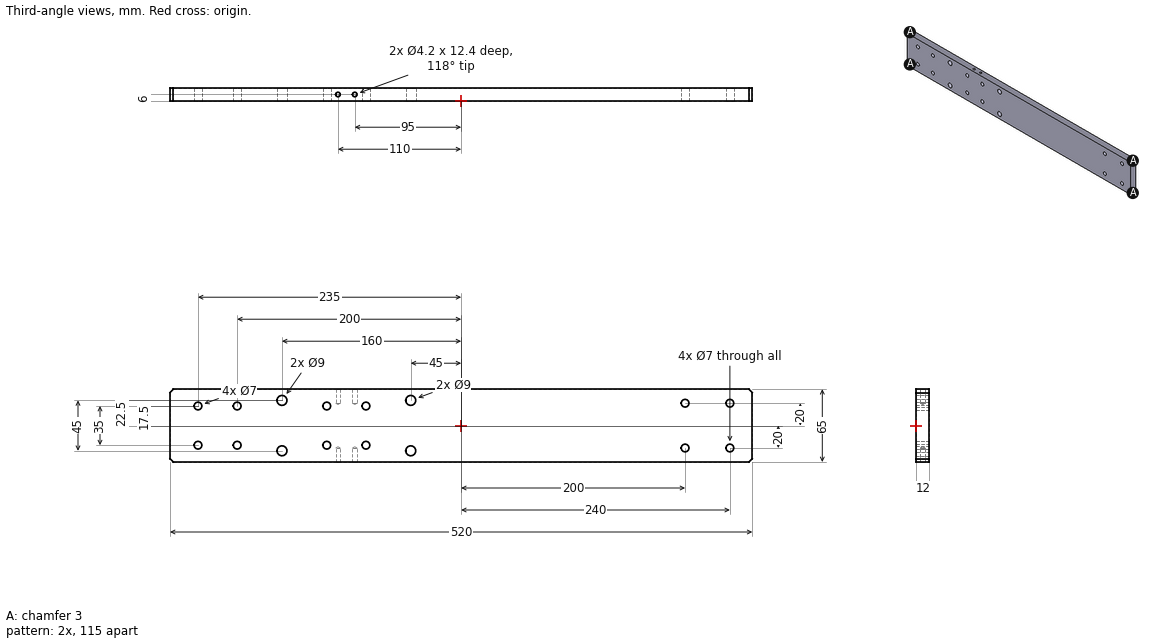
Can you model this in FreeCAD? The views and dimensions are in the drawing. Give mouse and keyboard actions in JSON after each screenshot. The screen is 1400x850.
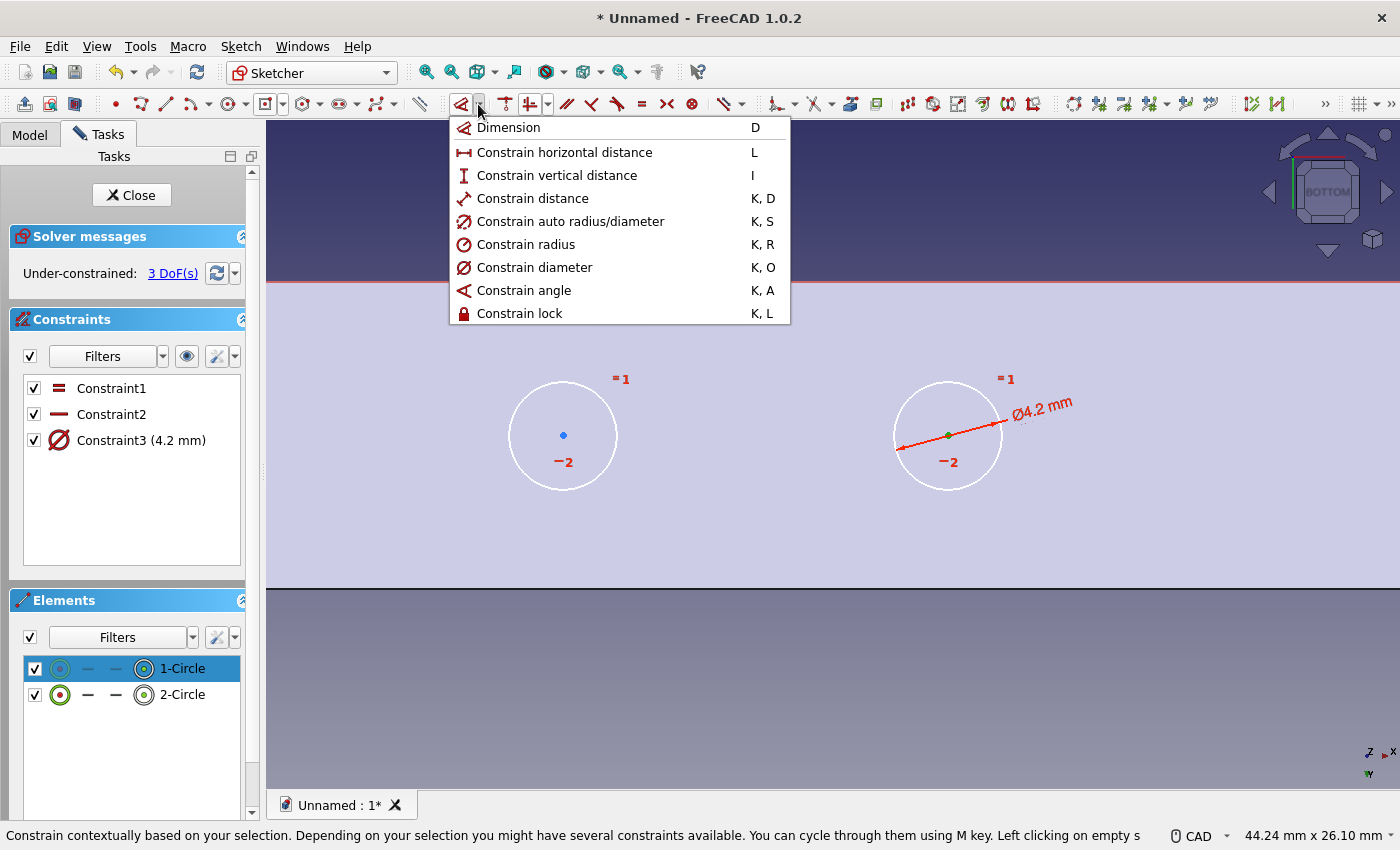
{"action": "left_click", "coordinate": [620, 176]}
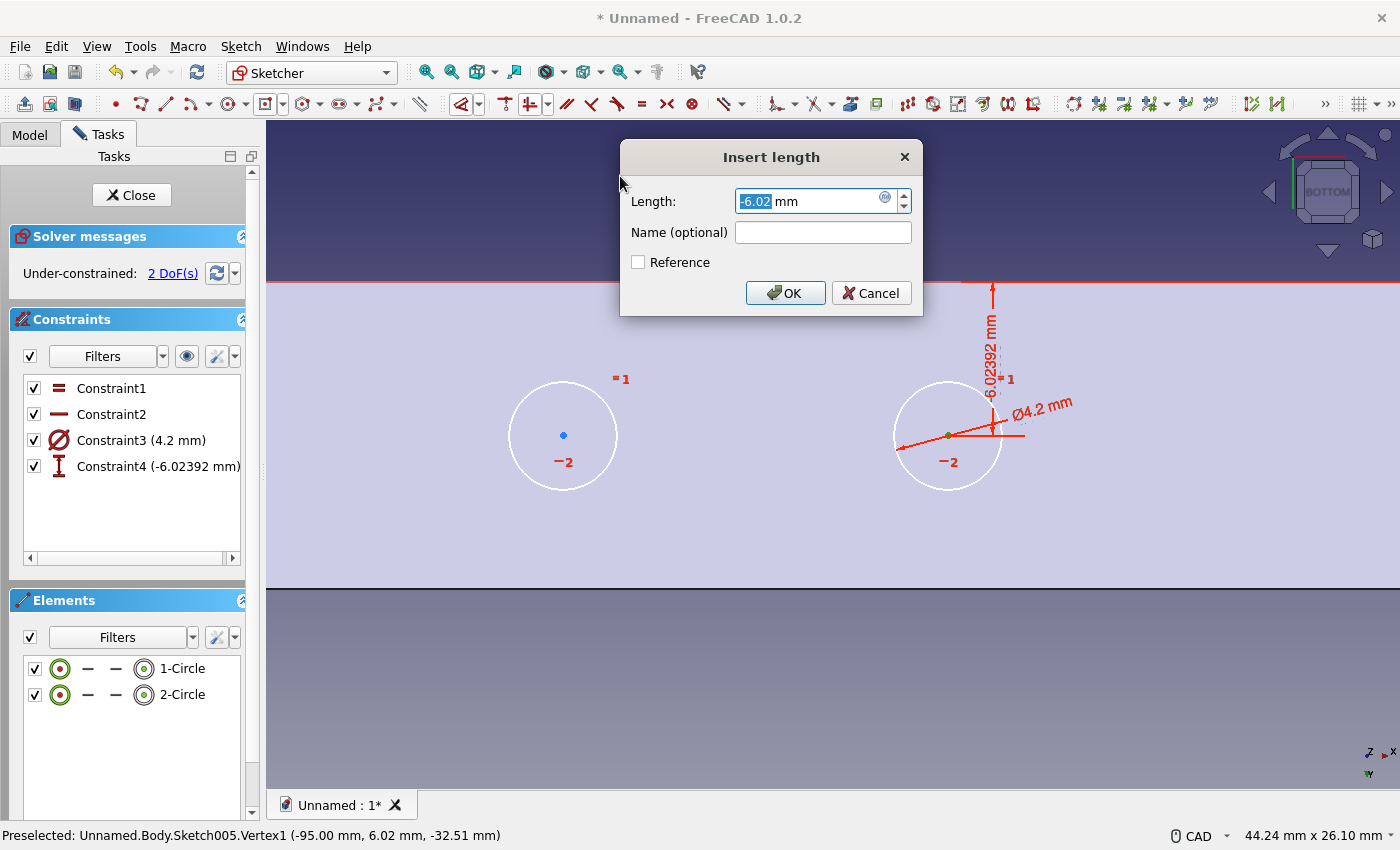
{"action": "type", "text": "-6"}
{"action": "key", "text": "Return"}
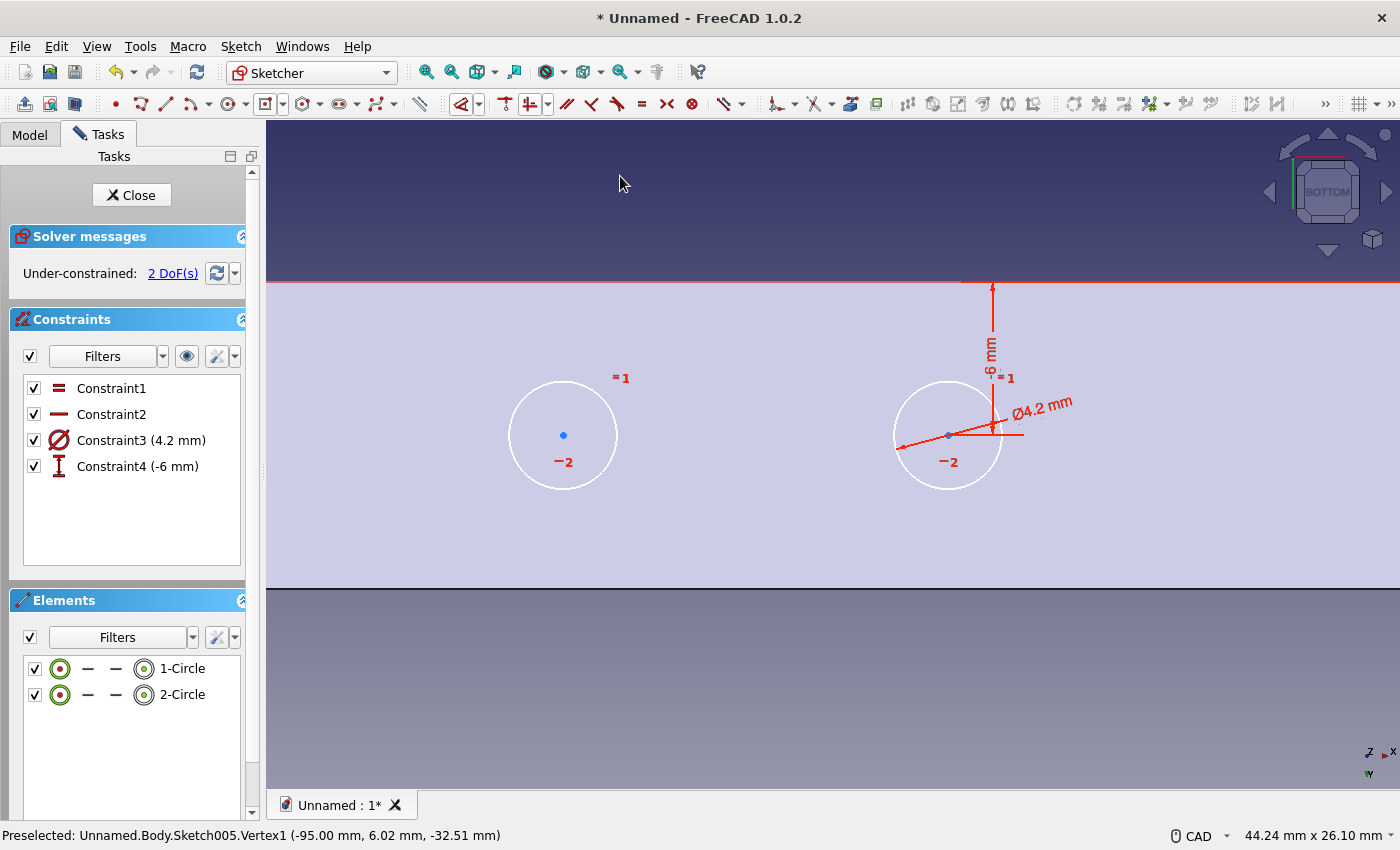
{"action": "left_click", "coordinate": [948, 435]}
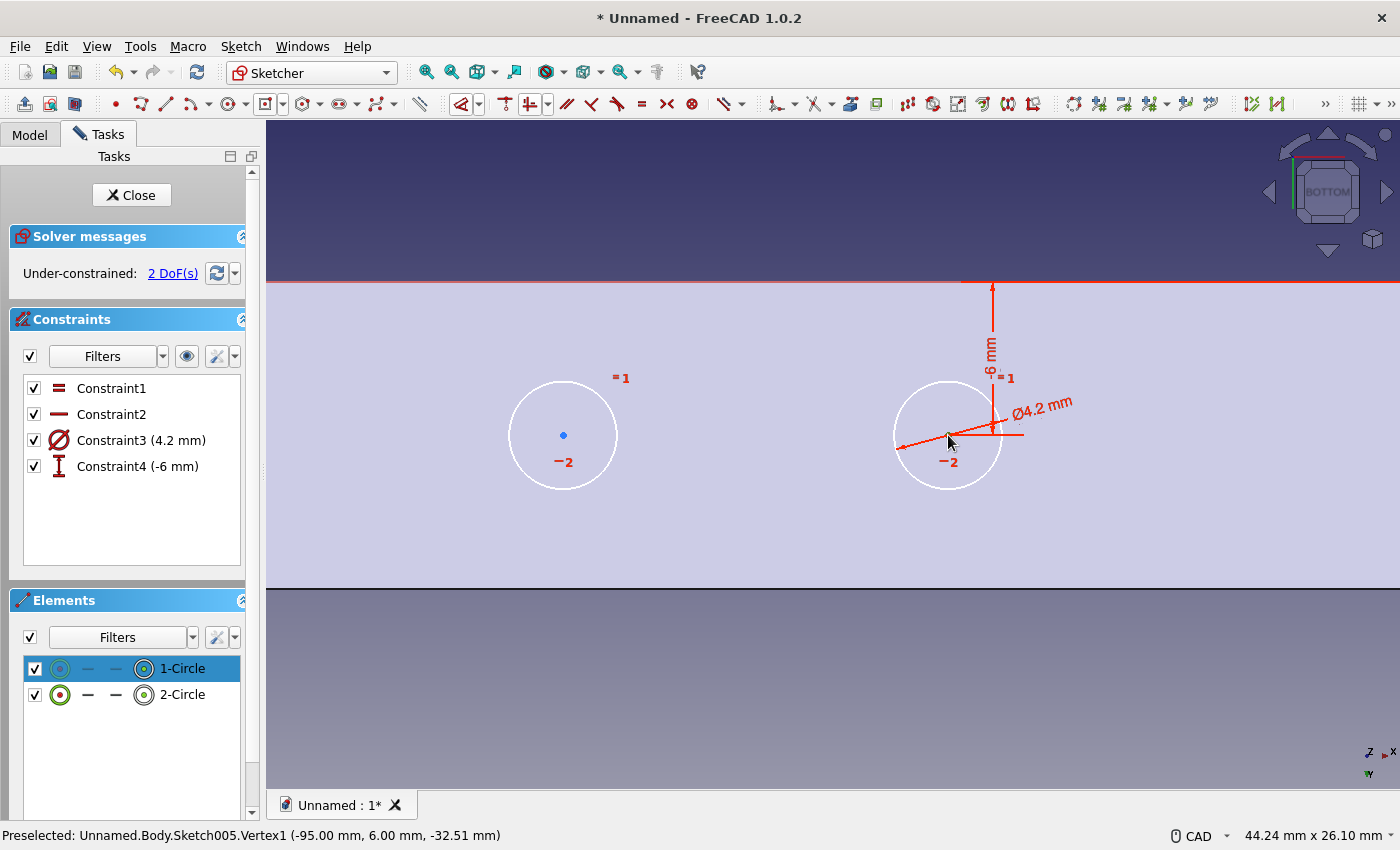
{"action": "key", "text": "l"}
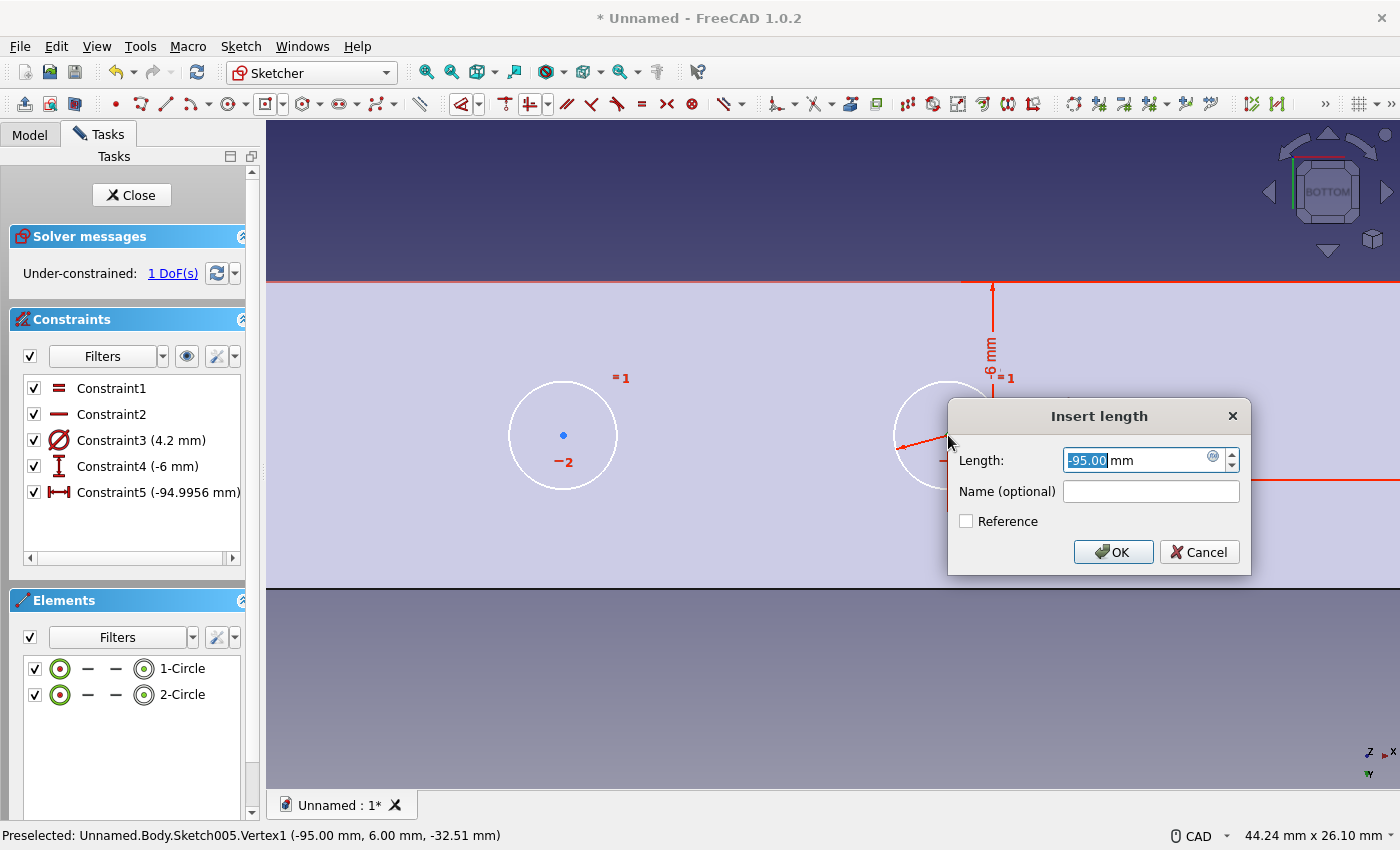
{"action": "type", "text": "-95"}
{"action": "key", "text": "Return"}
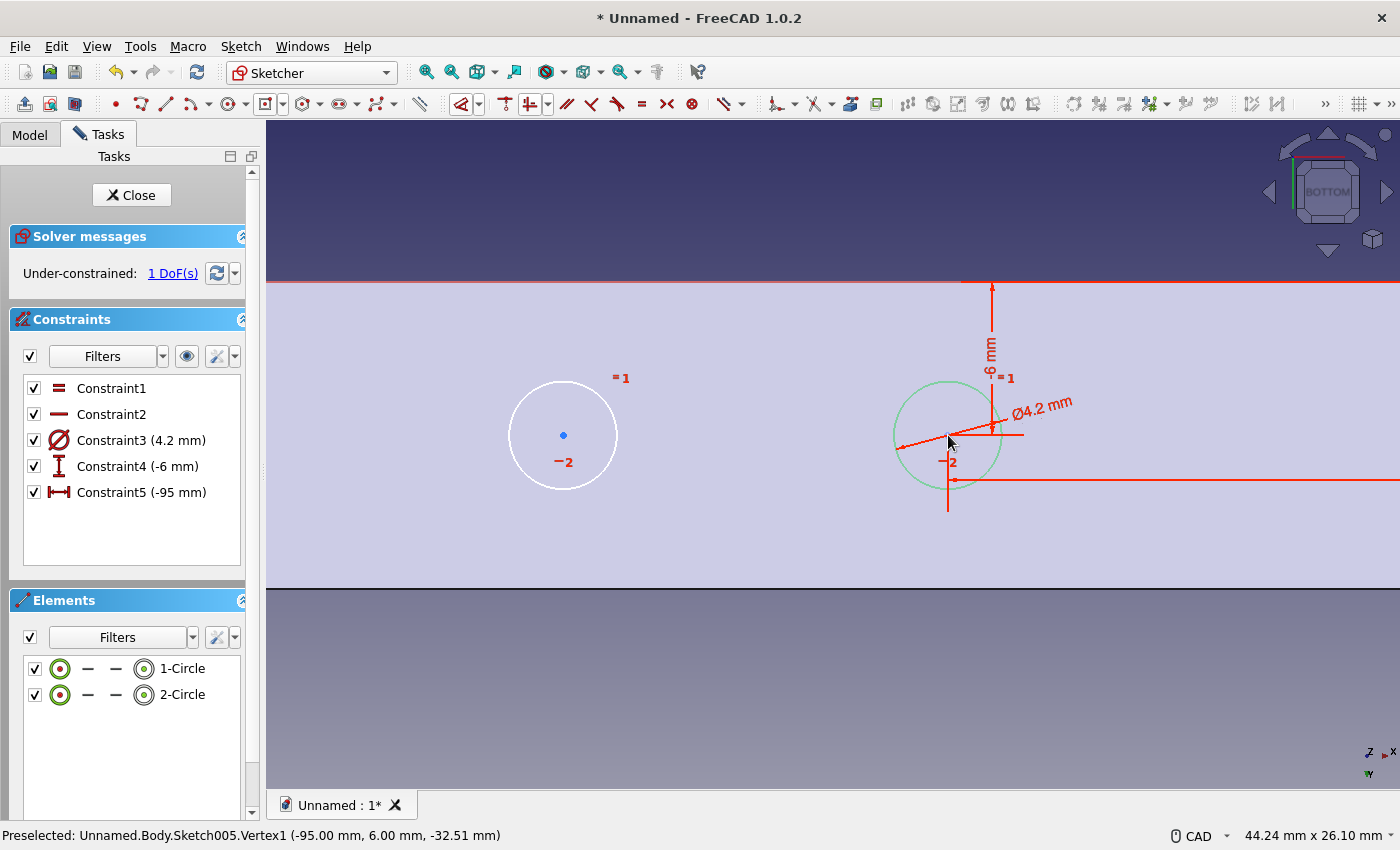
{"action": "left_click", "coordinate": [563, 435]}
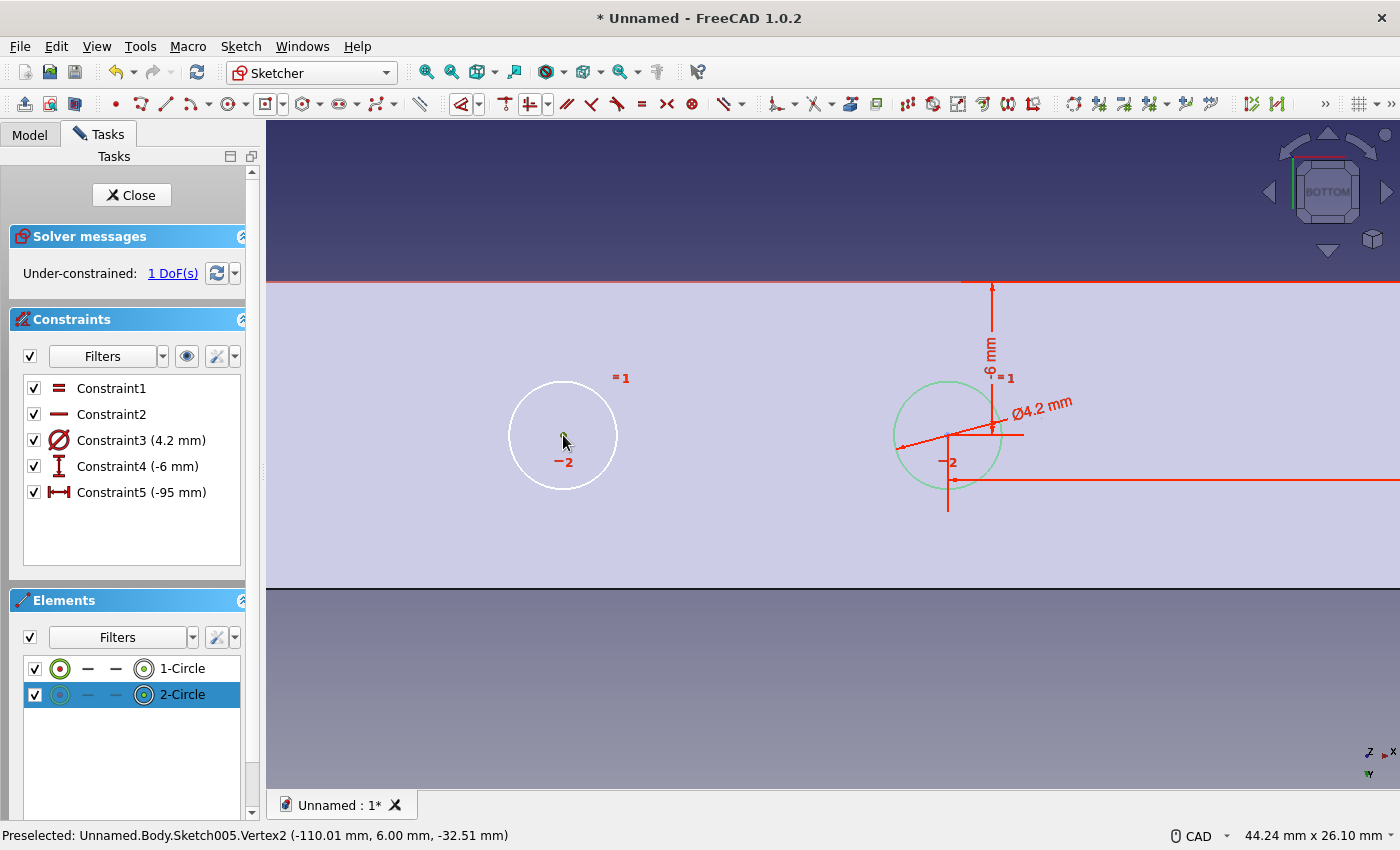
{"action": "key", "text": "l"}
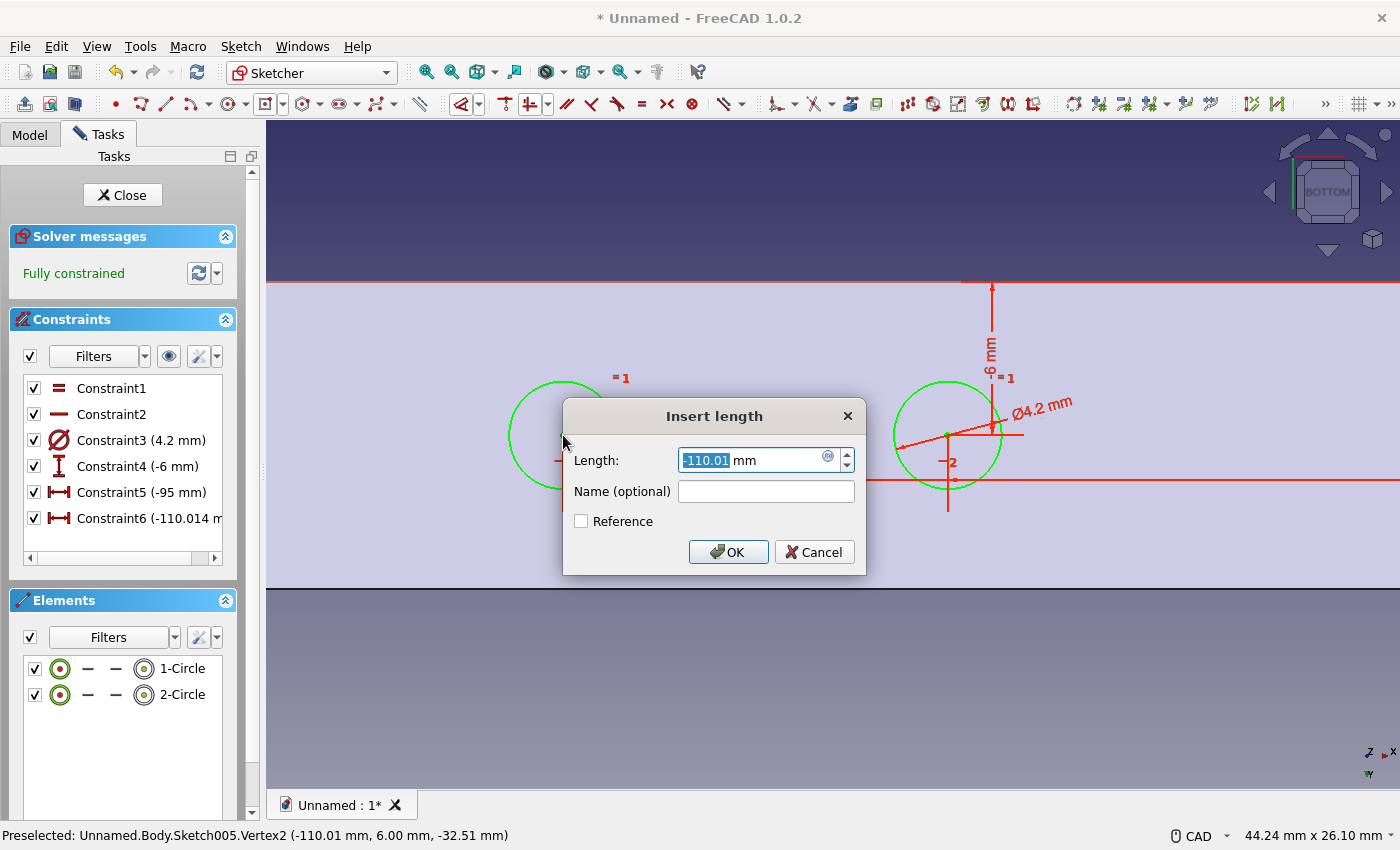
{"action": "type", "text": "-110"}
{"action": "key", "text": "Return"}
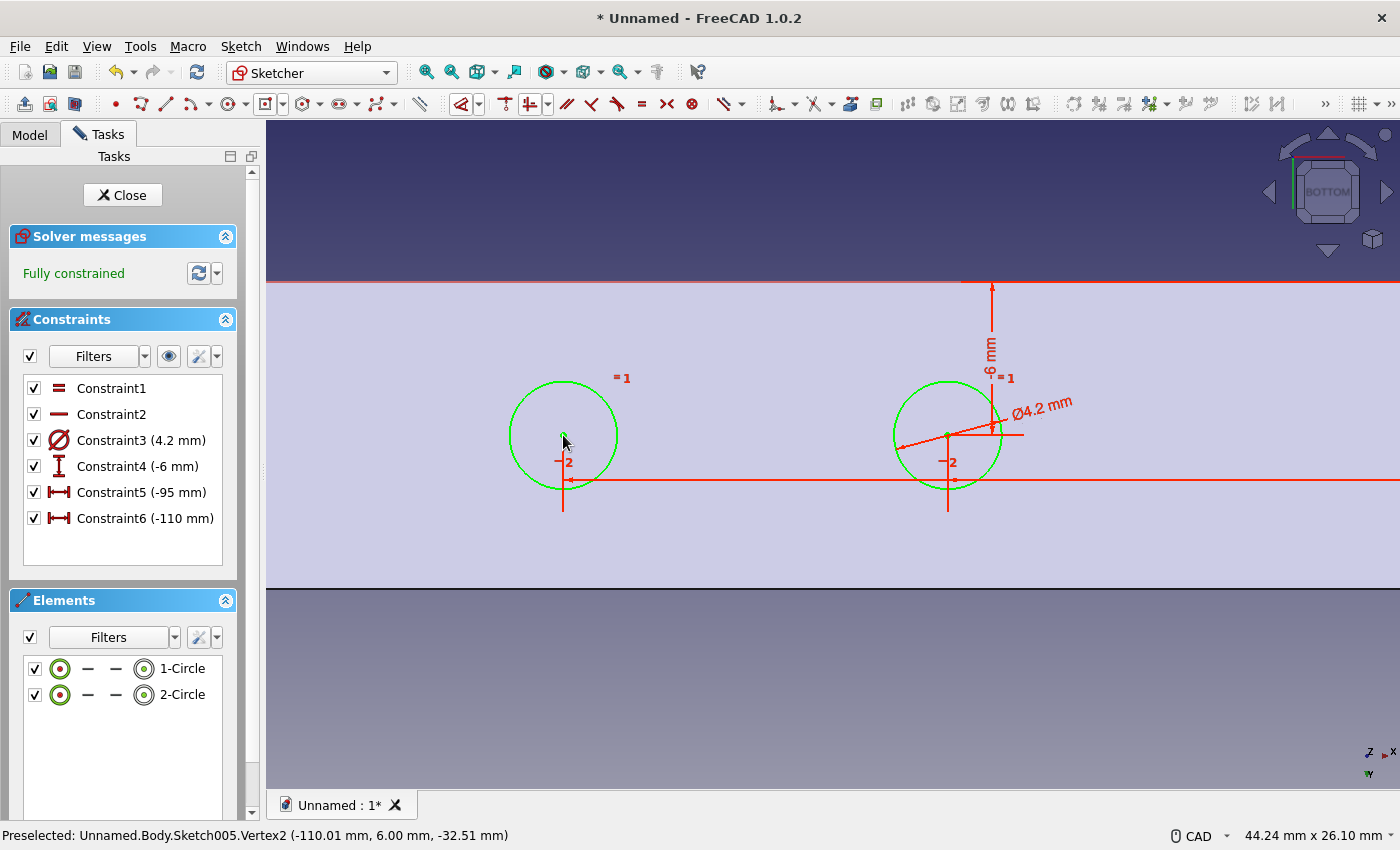
{"action": "left_click", "coordinate": [123, 195]}